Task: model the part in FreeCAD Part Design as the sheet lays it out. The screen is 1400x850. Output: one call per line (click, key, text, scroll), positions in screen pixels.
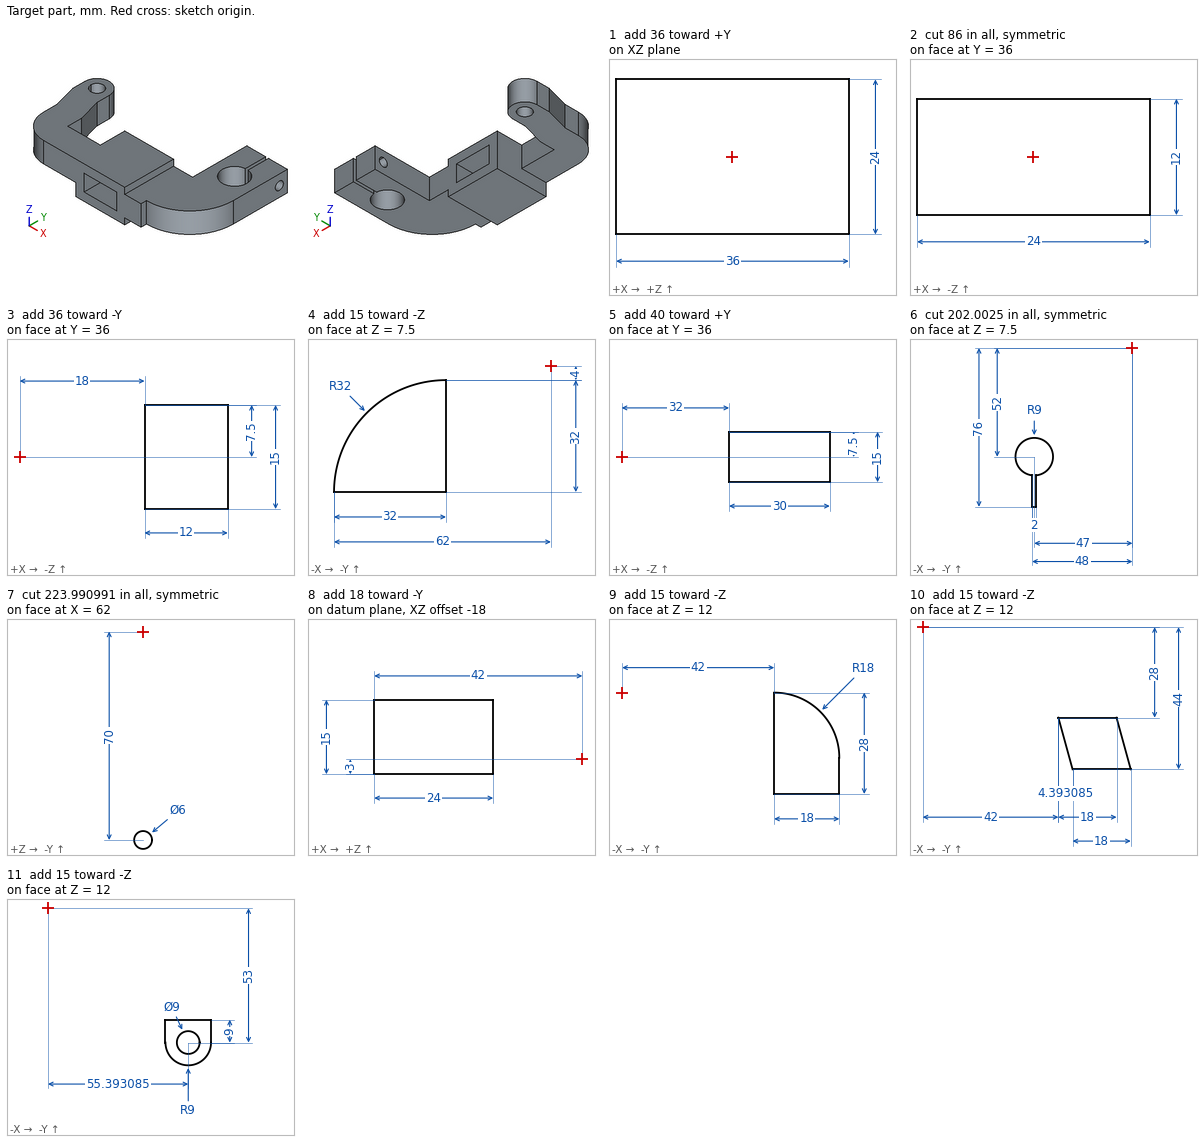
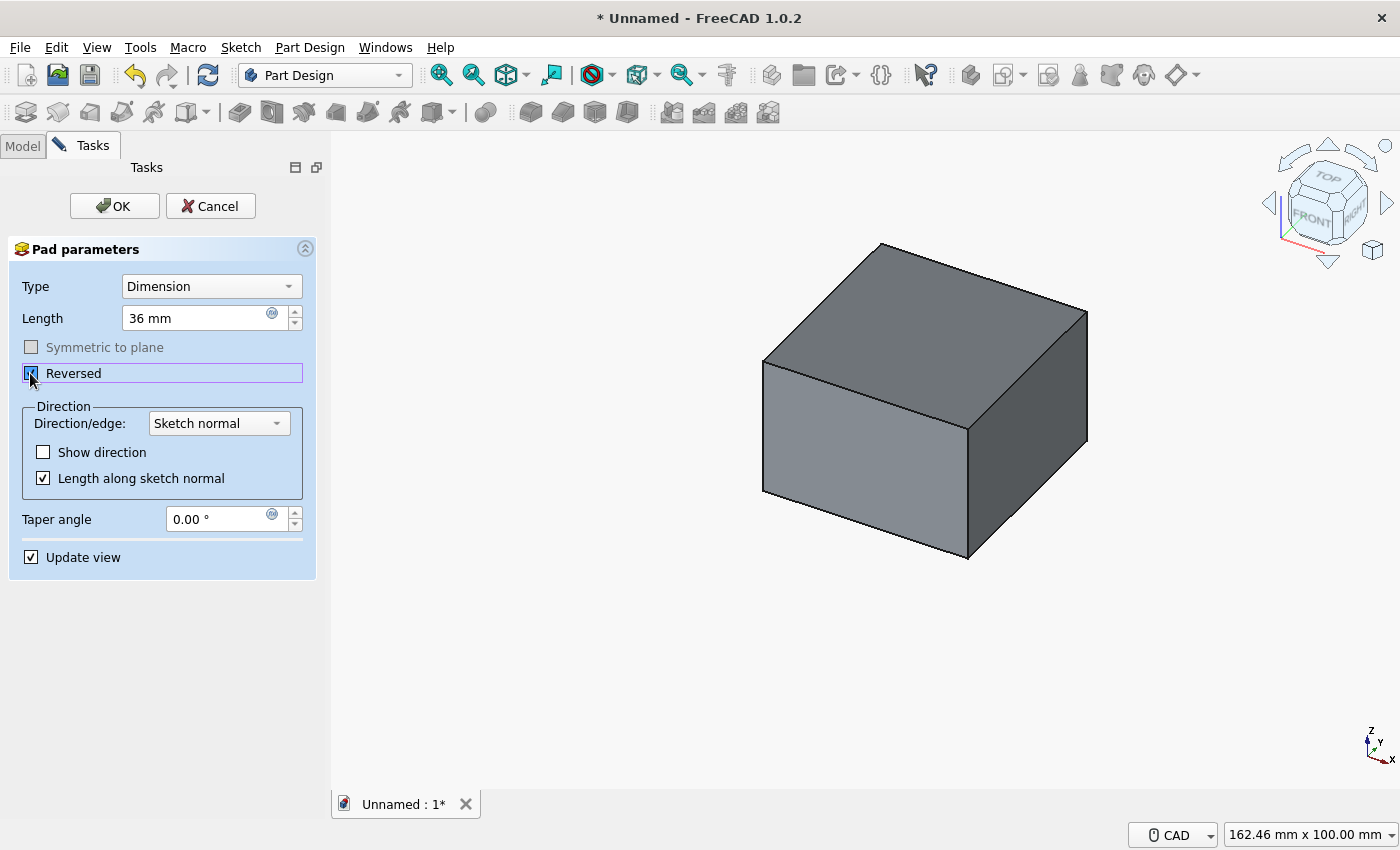
click(115, 206)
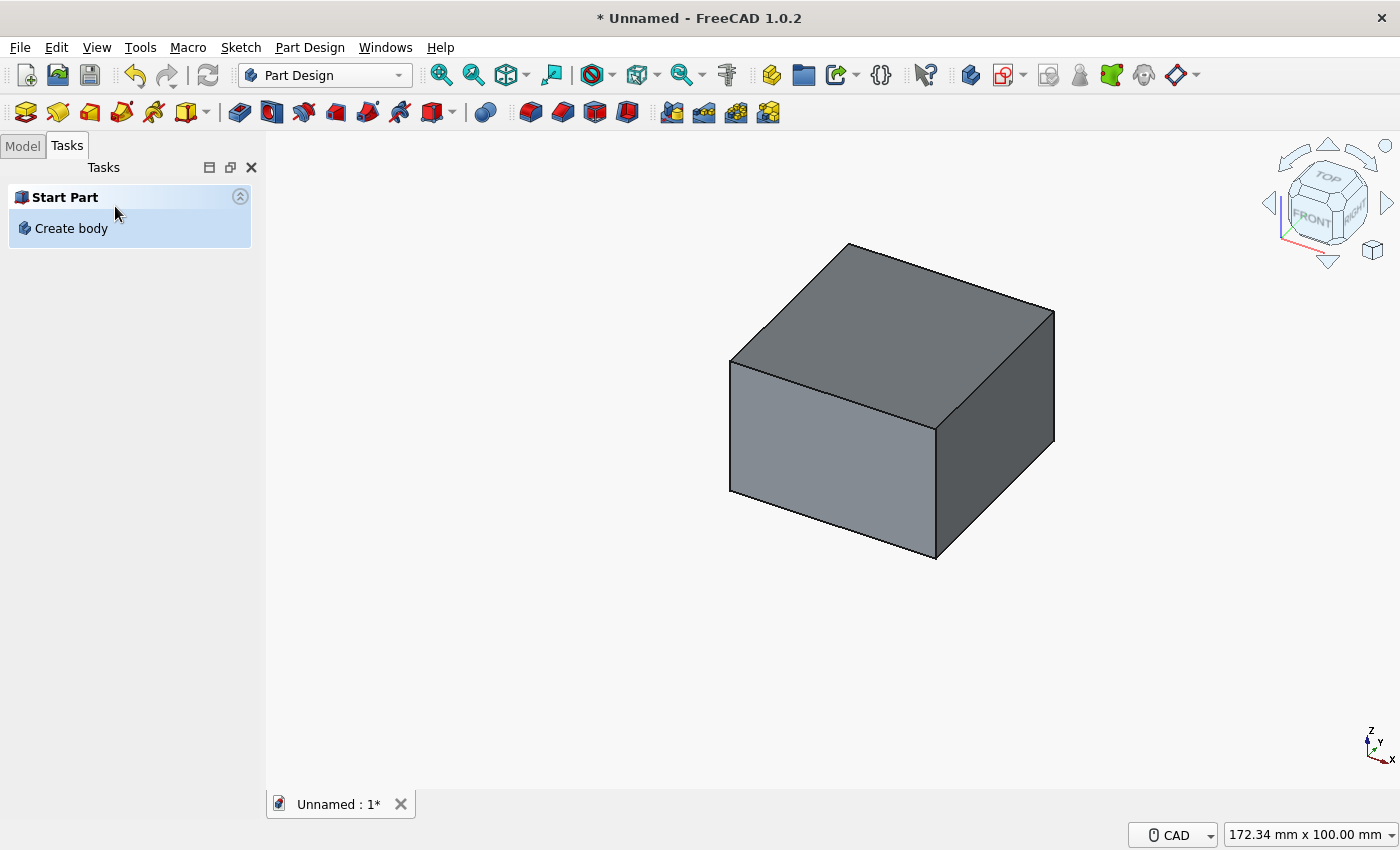
key(4)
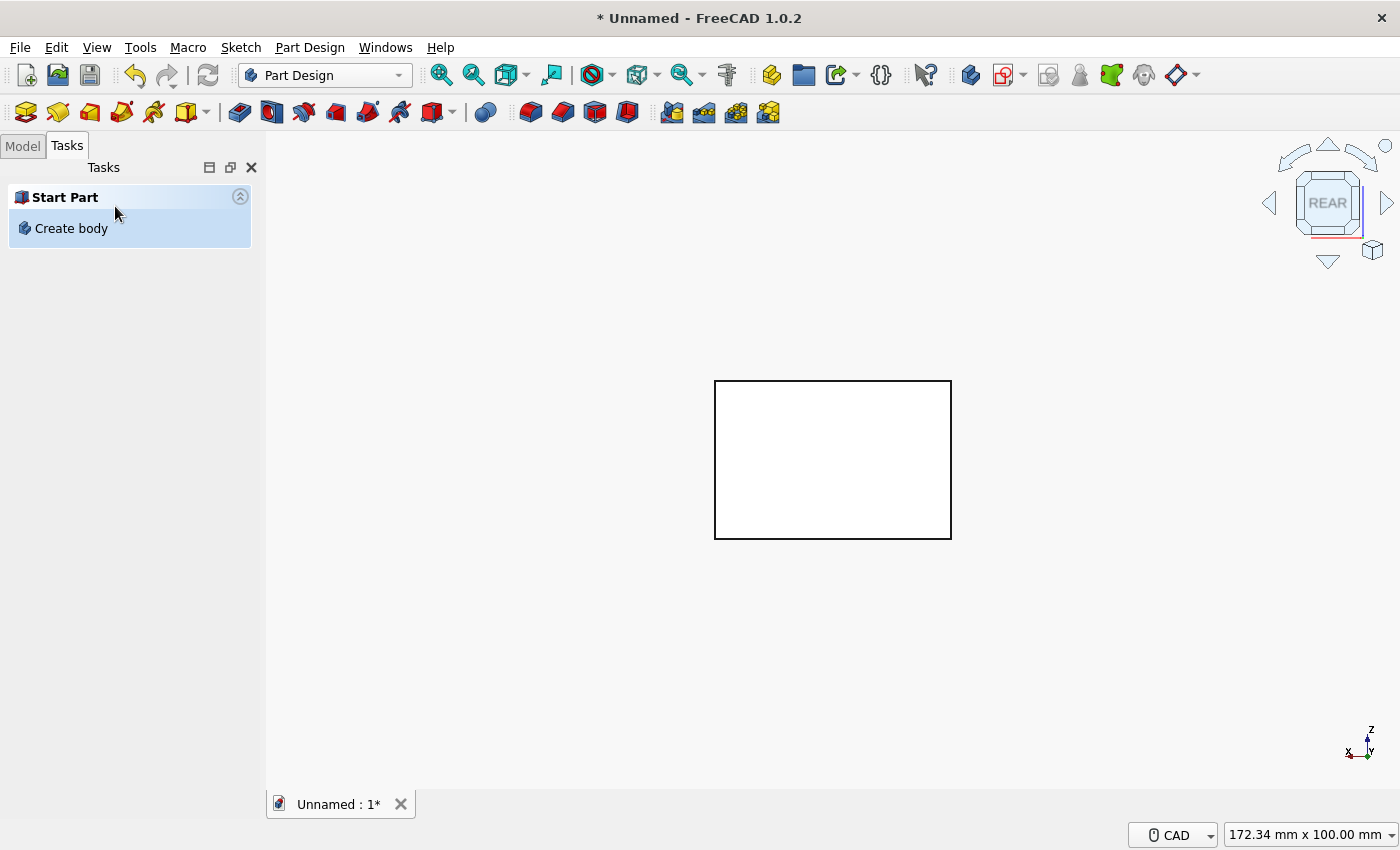
click(442, 76)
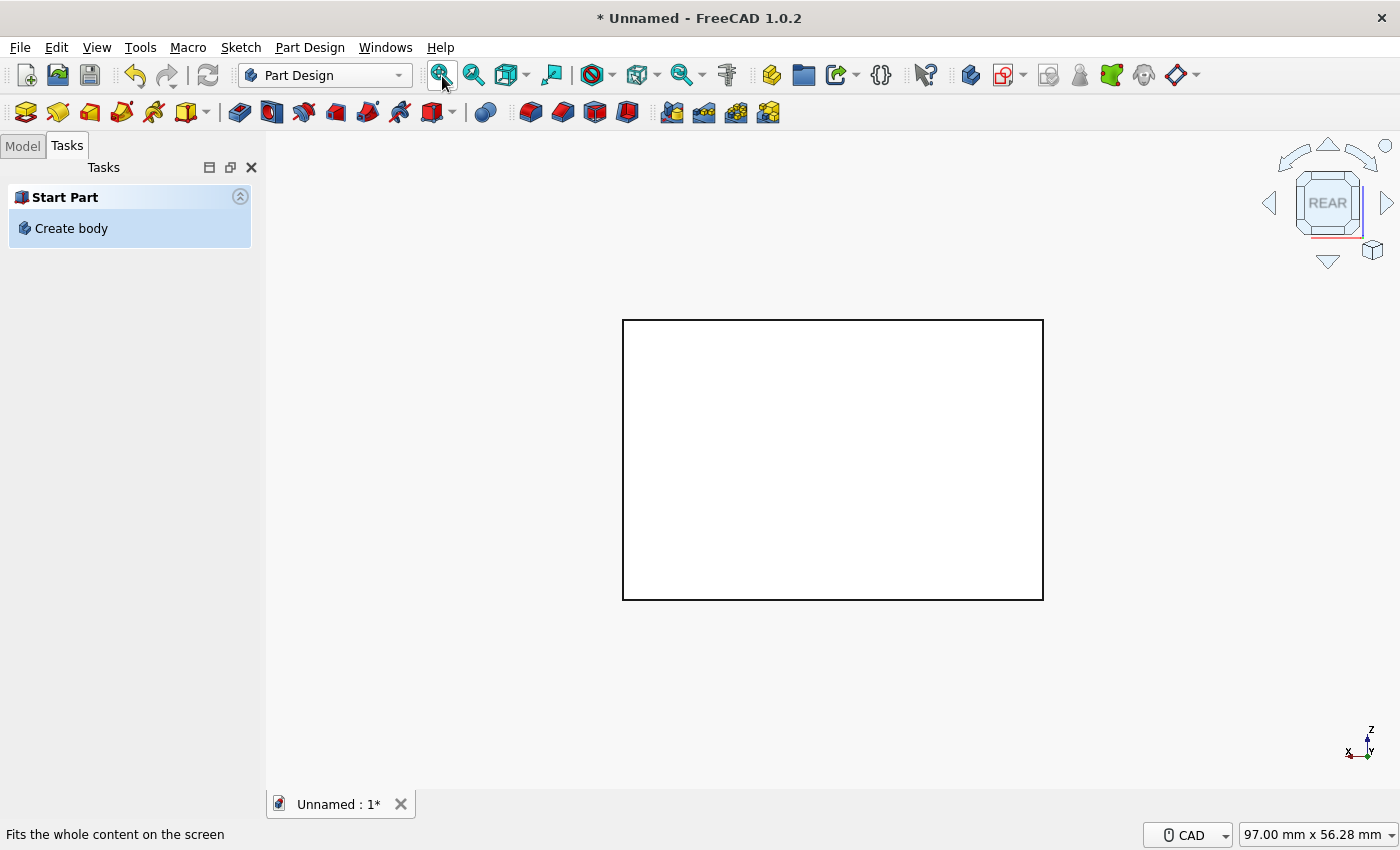
click(773, 459)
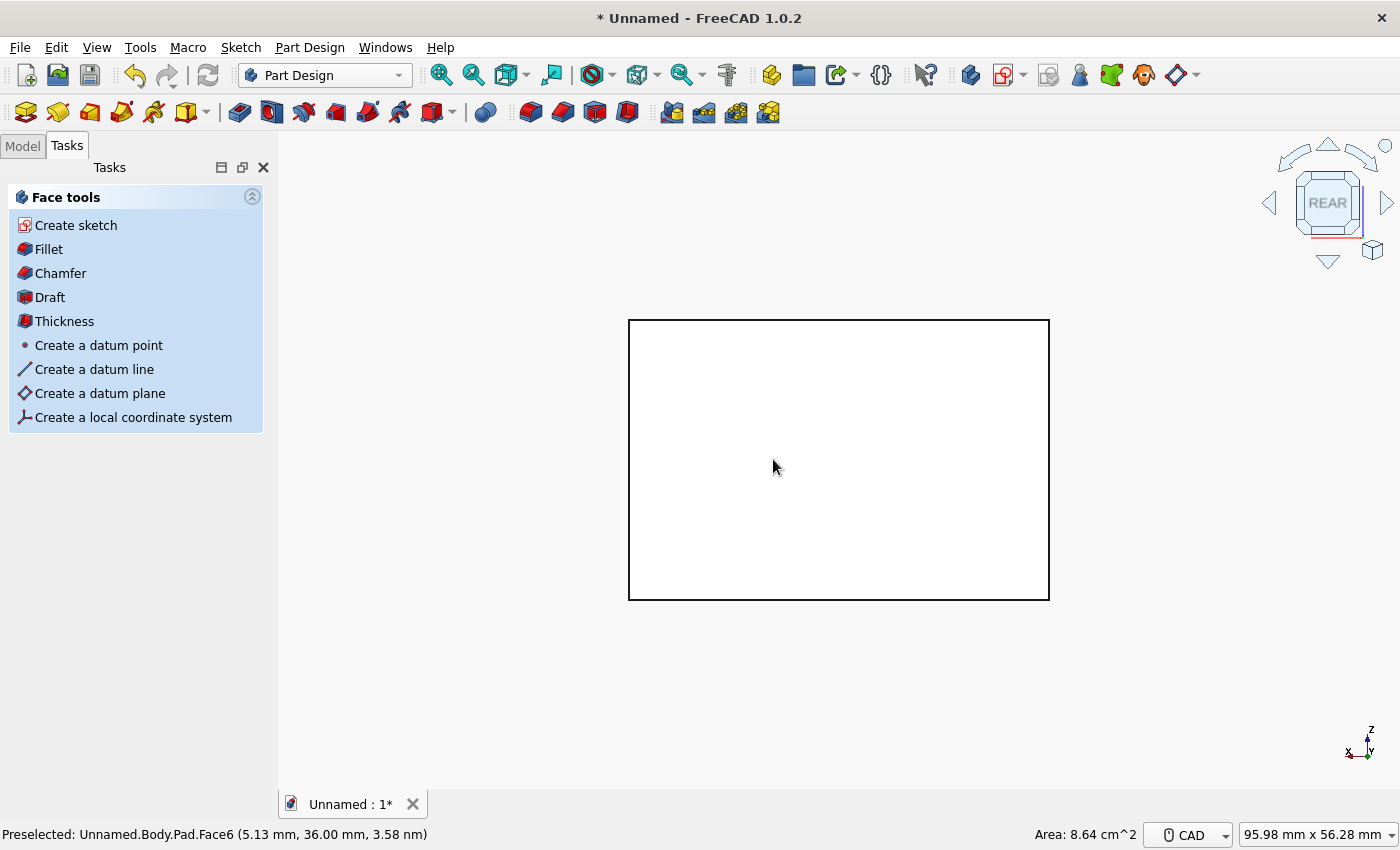
click(1004, 76)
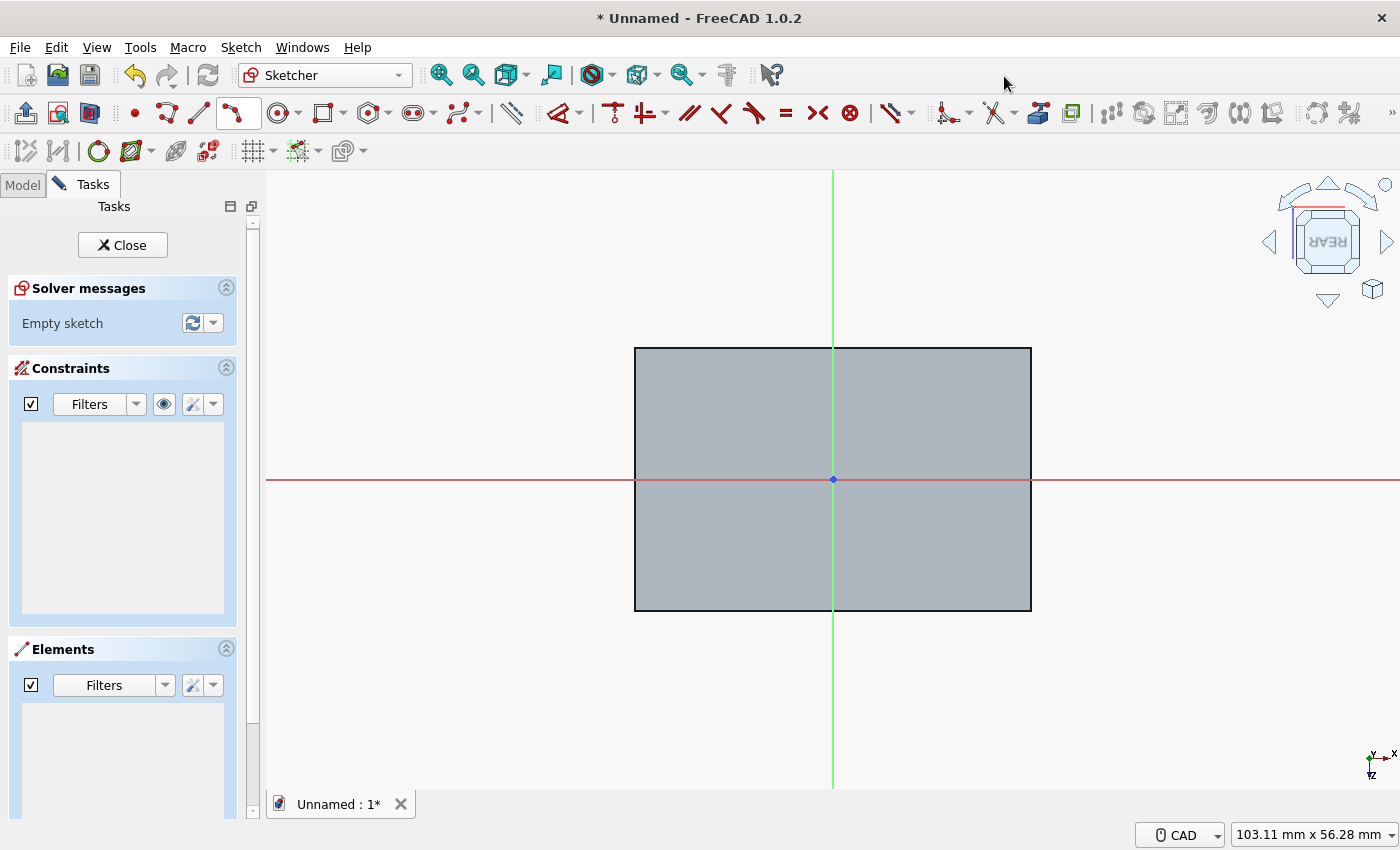
scroll(873, 479, up, 5)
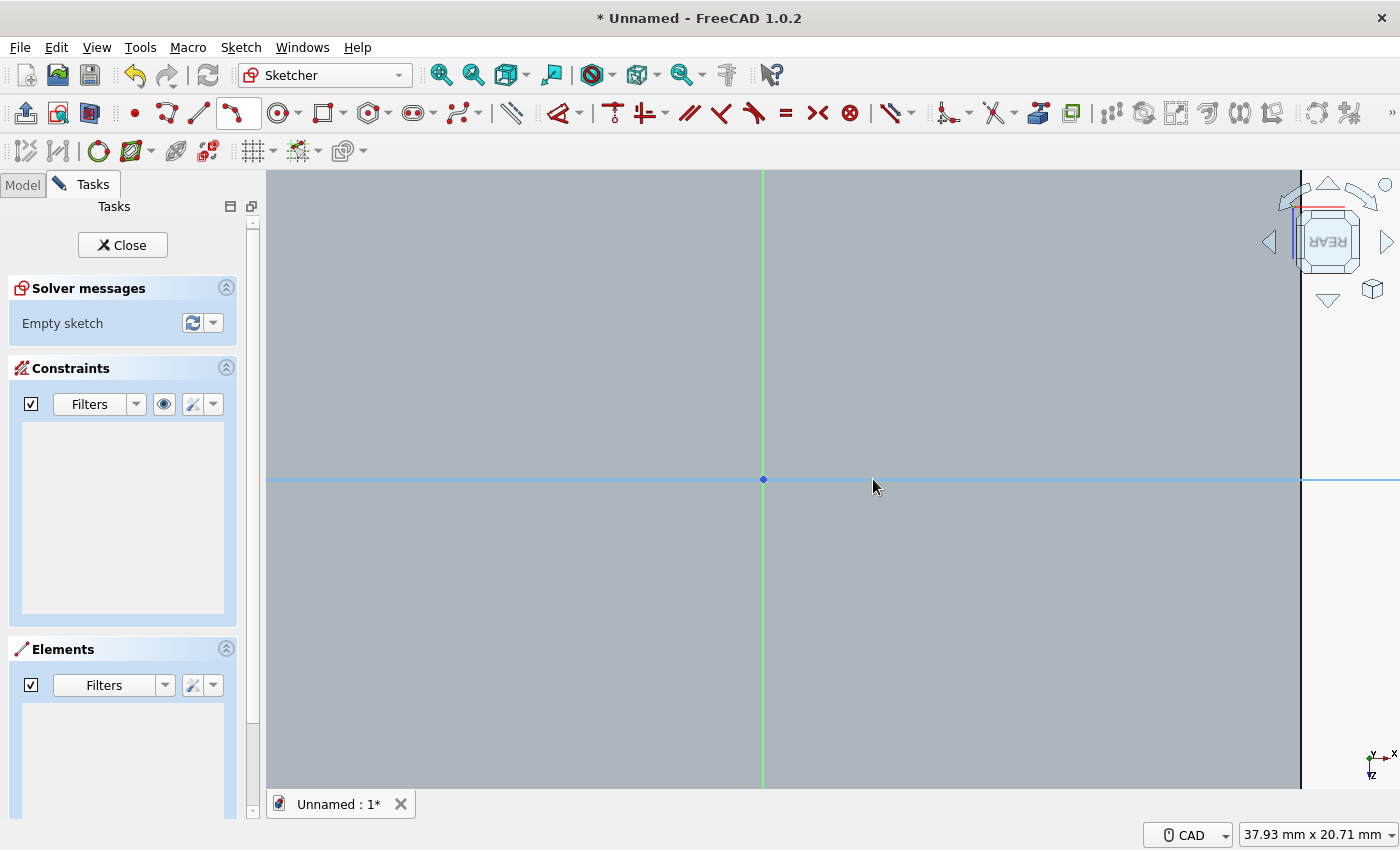
key(g)
key(v)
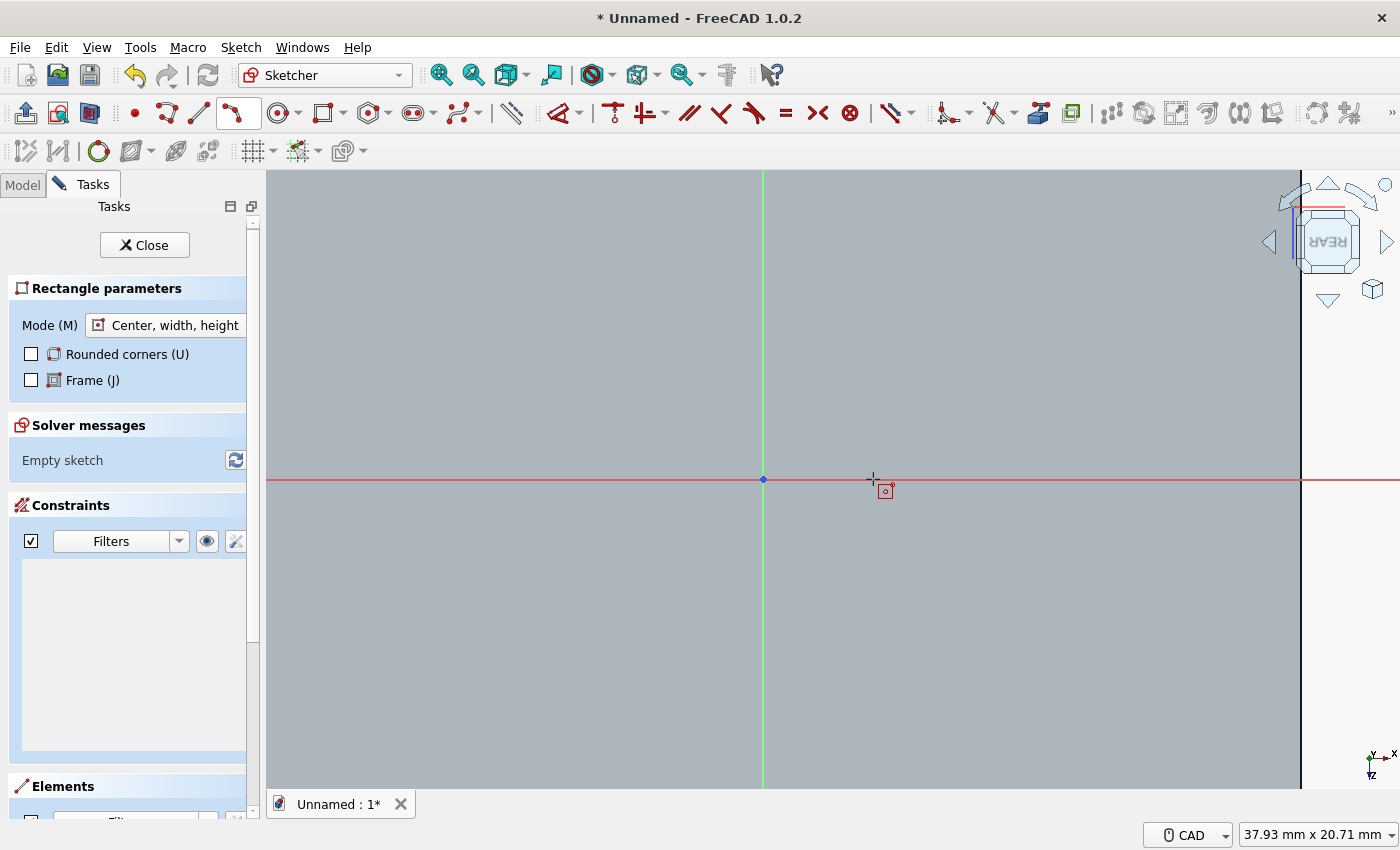
click(763, 479)
click(1122, 300)
key(Escape)